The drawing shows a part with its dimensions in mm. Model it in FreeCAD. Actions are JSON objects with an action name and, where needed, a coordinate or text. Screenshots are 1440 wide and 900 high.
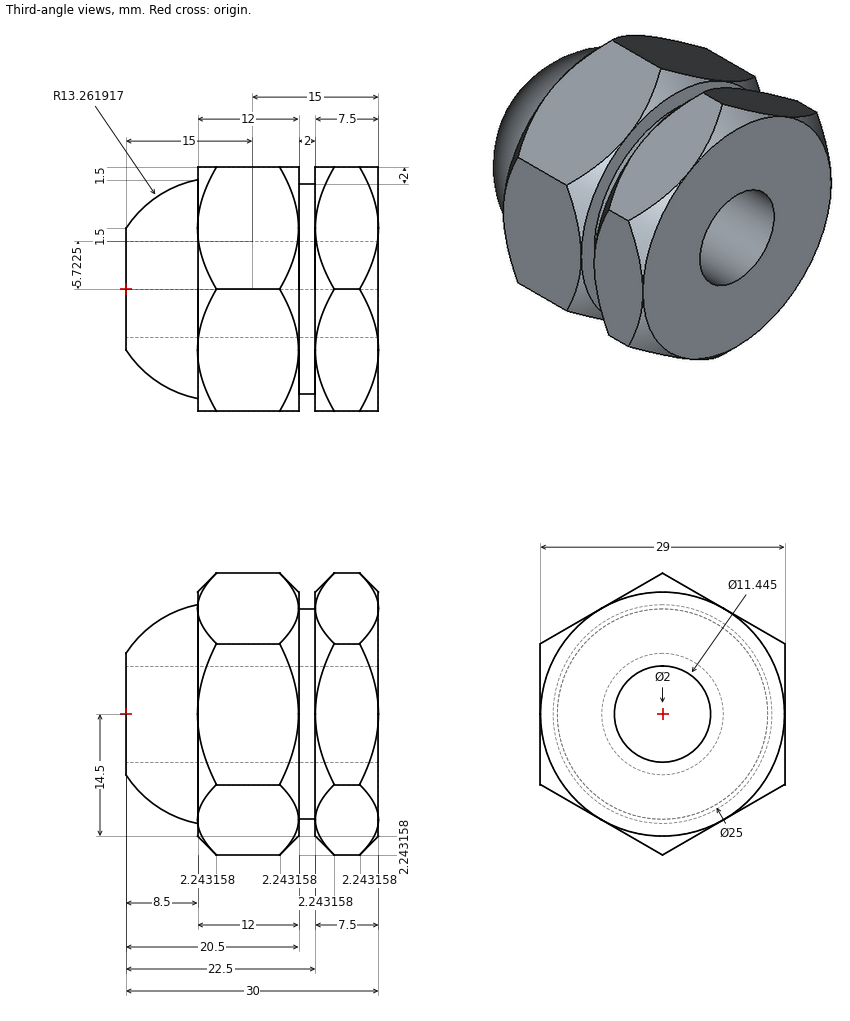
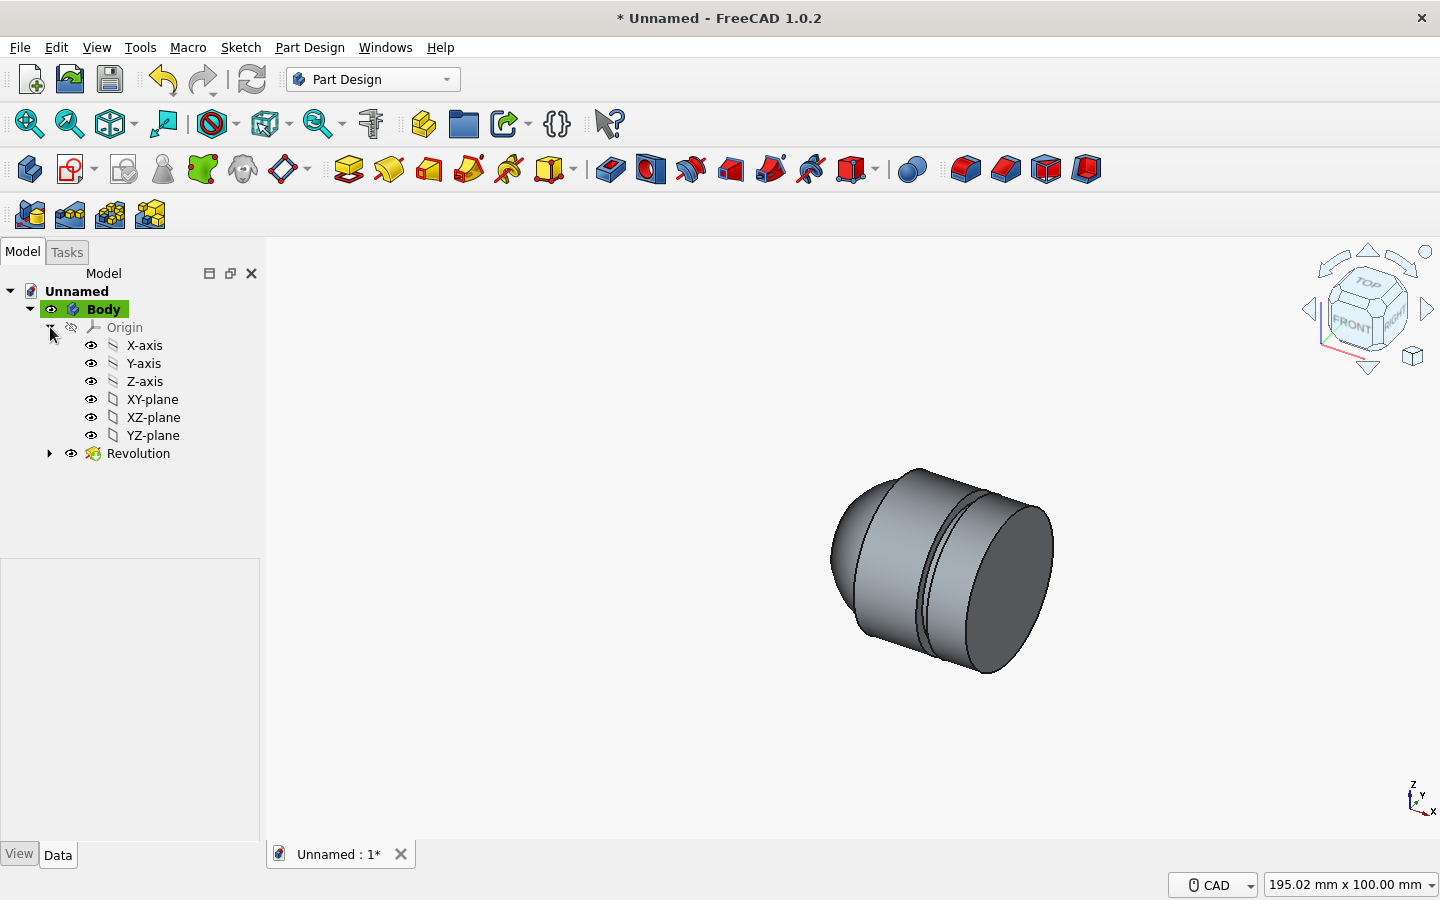
{"action": "left_click", "coordinate": [136, 435]}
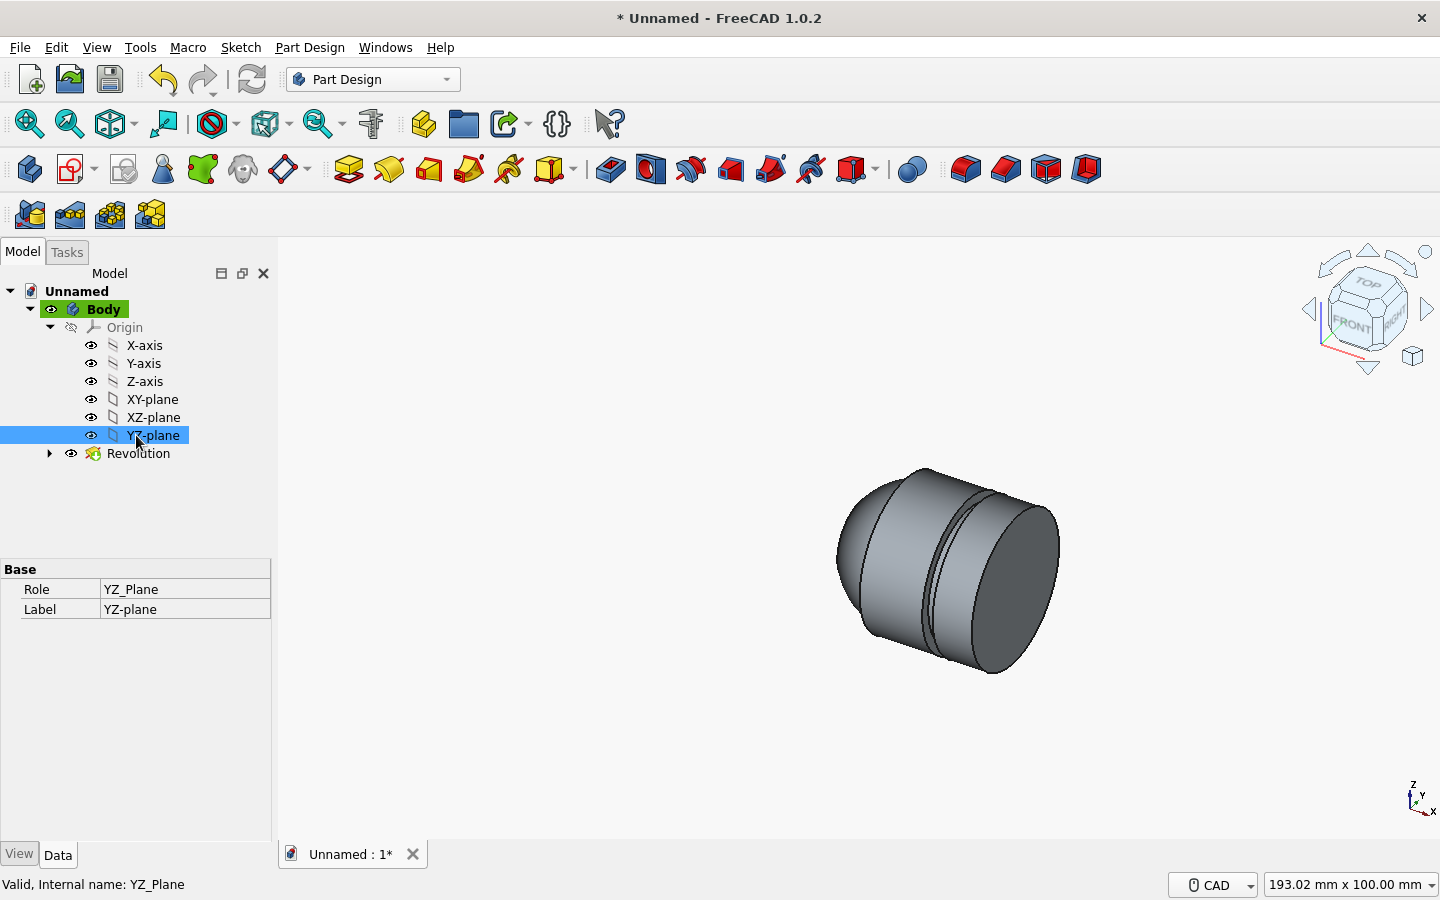
{"action": "left_click", "coordinate": [284, 170]}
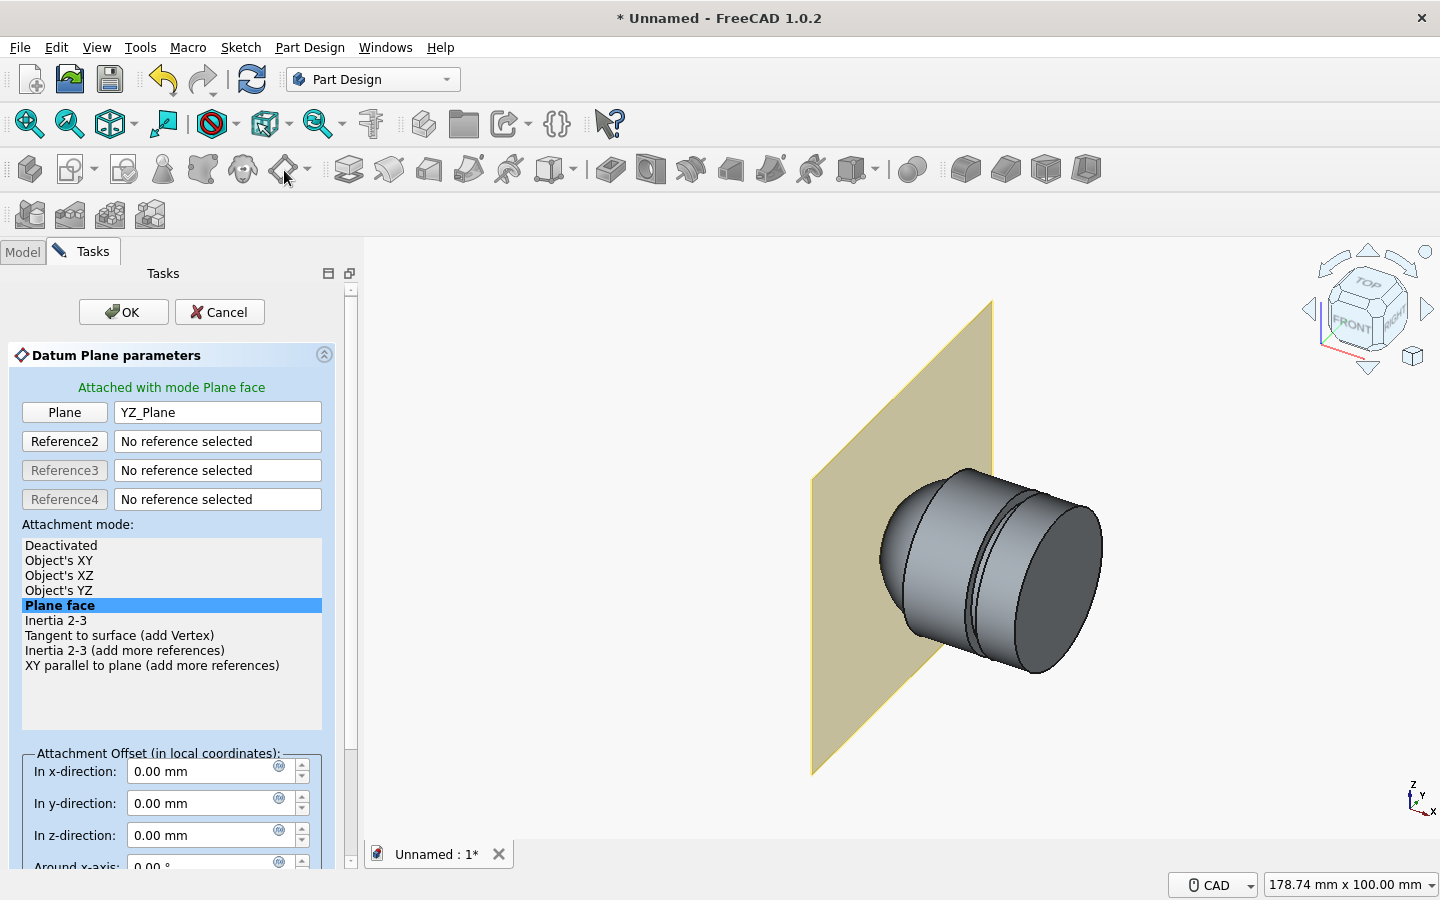
{"action": "triple_click", "coordinate": [210, 835]}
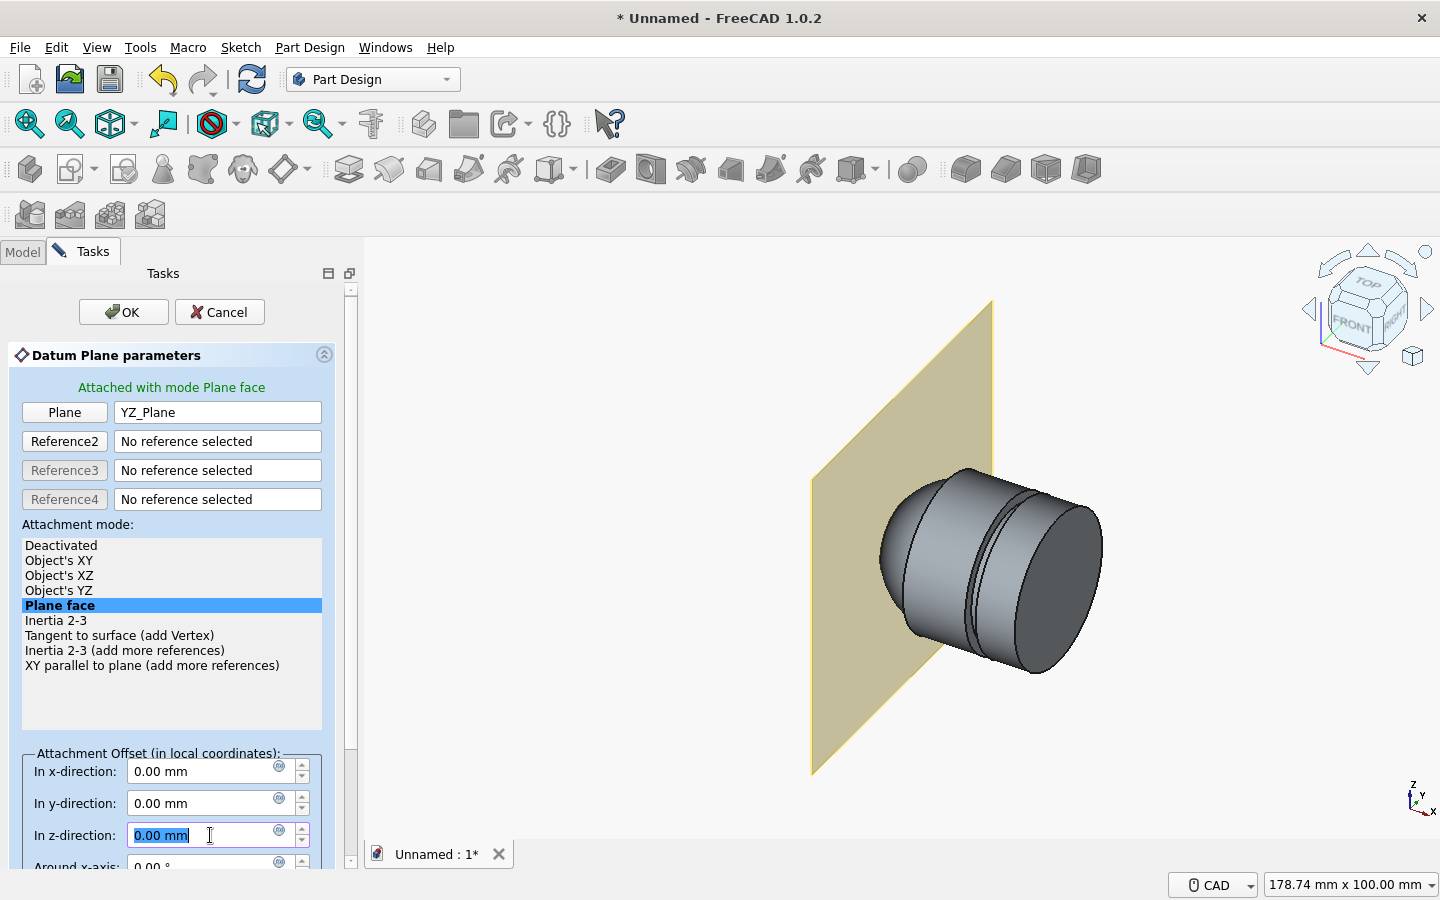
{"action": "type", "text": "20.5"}
{"action": "key", "text": "Tab"}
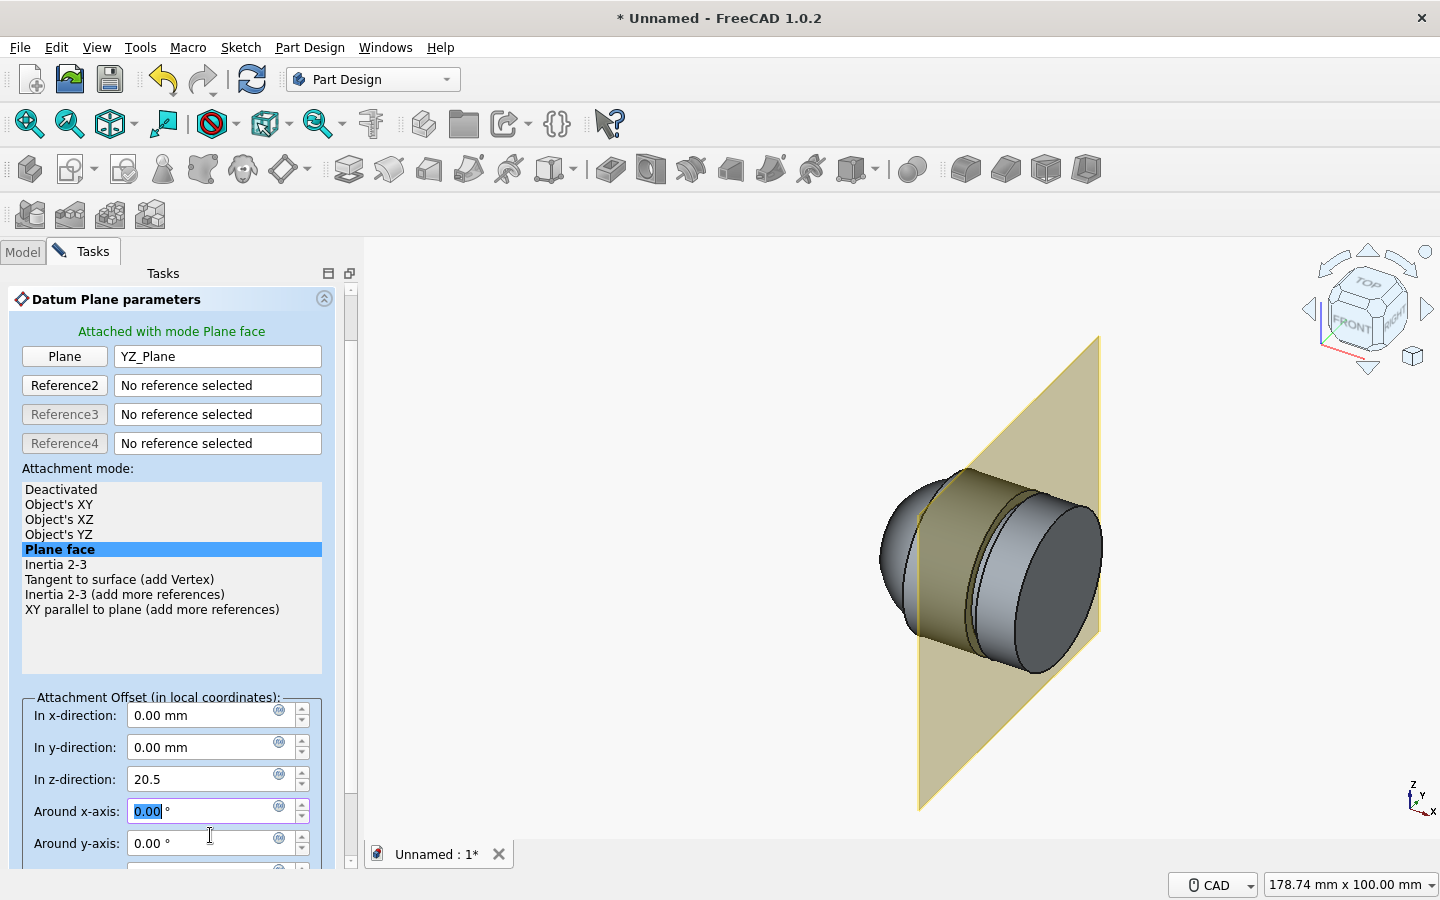
{"action": "scroll", "coordinate": [351, 576], "scroll_direction": "up", "scroll_amount": 2}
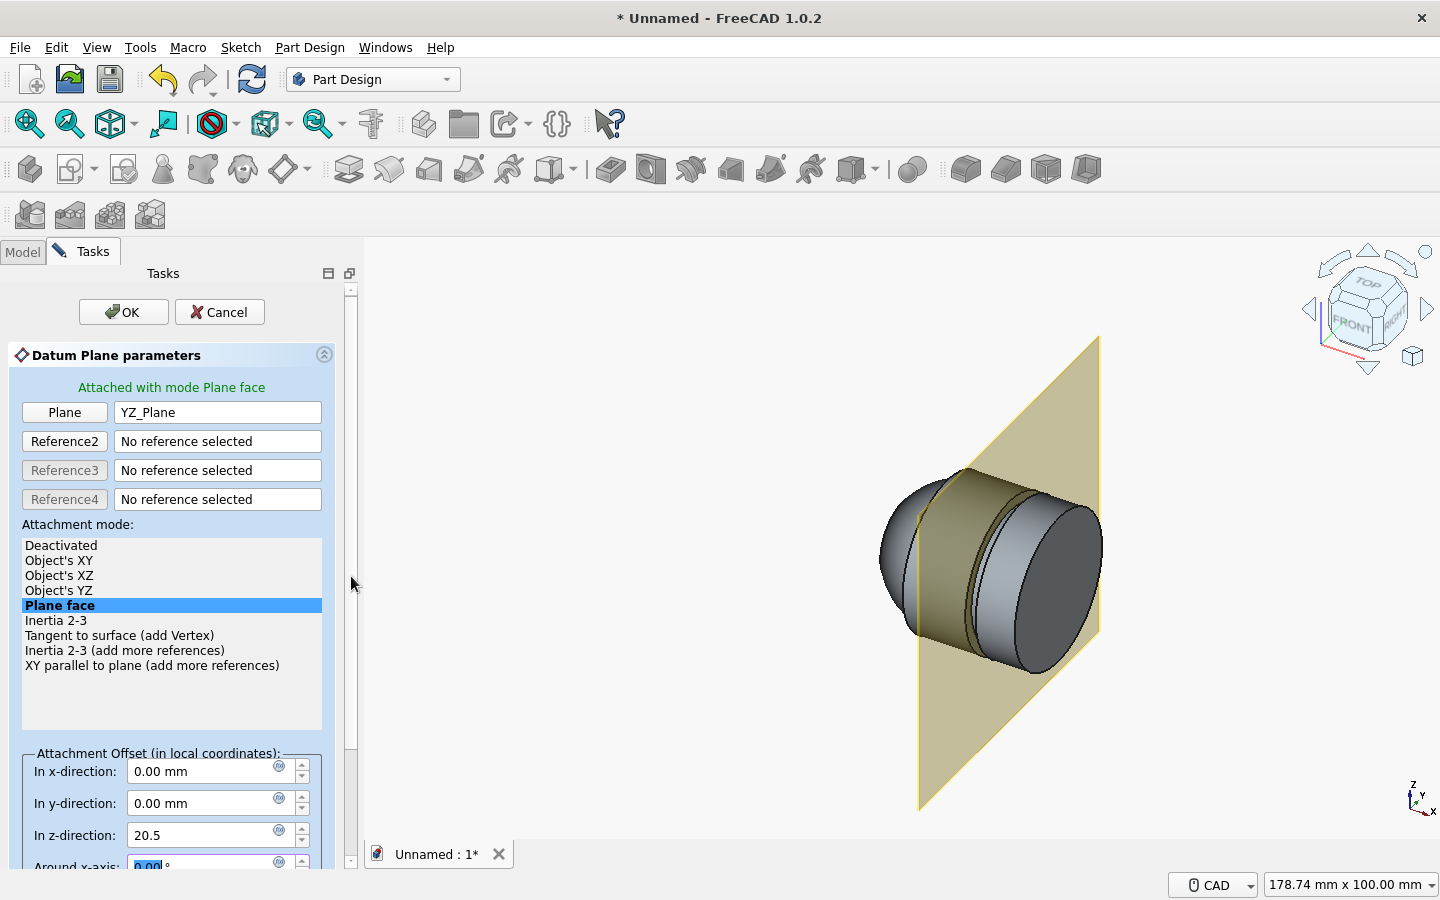
{"action": "left_click", "coordinate": [124, 312]}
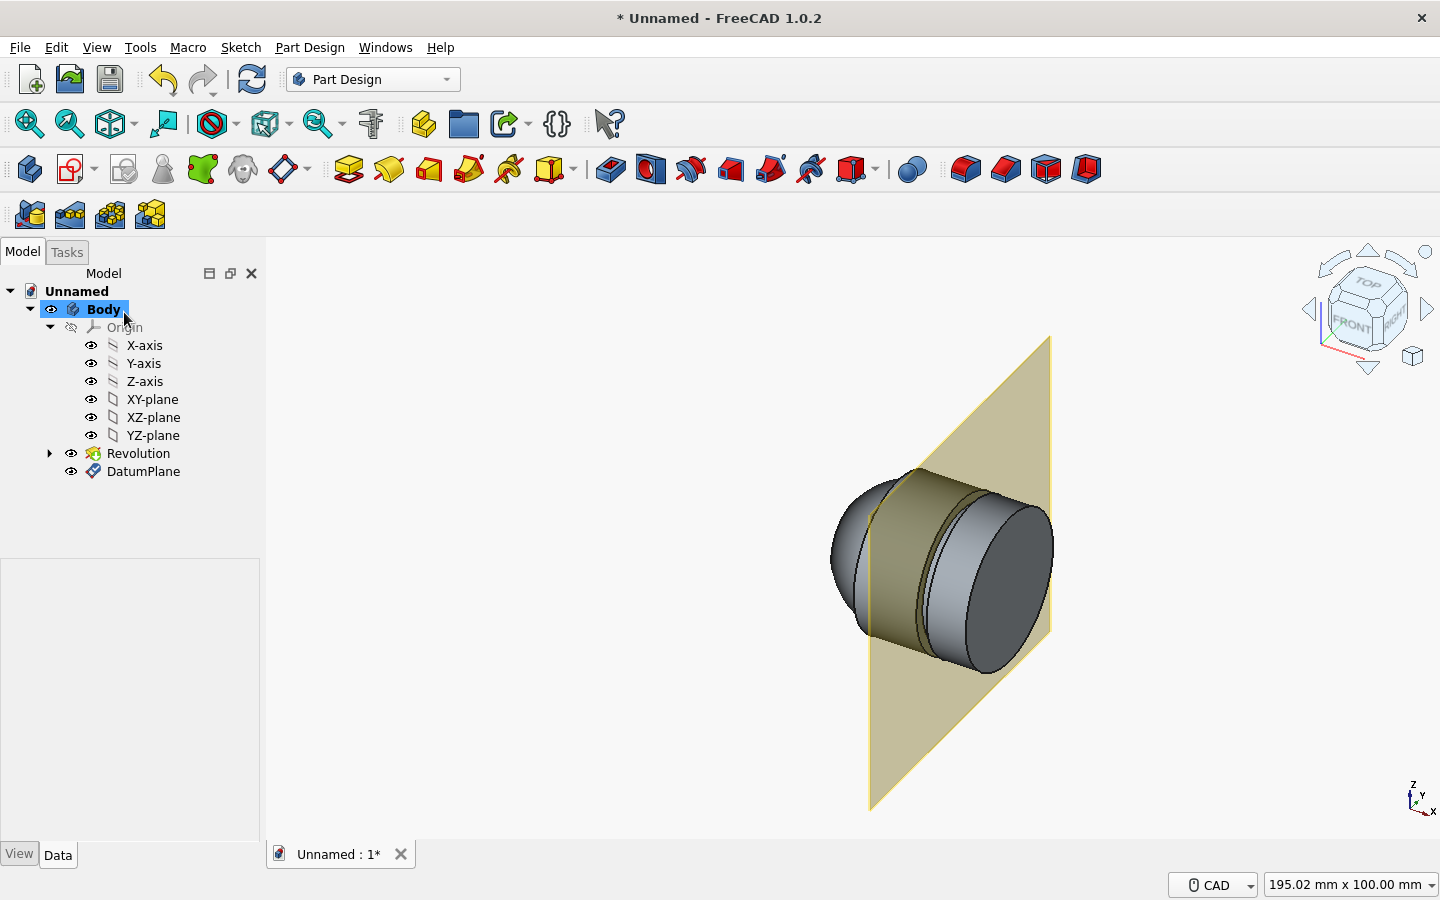
{"action": "left_click", "coordinate": [116, 471]}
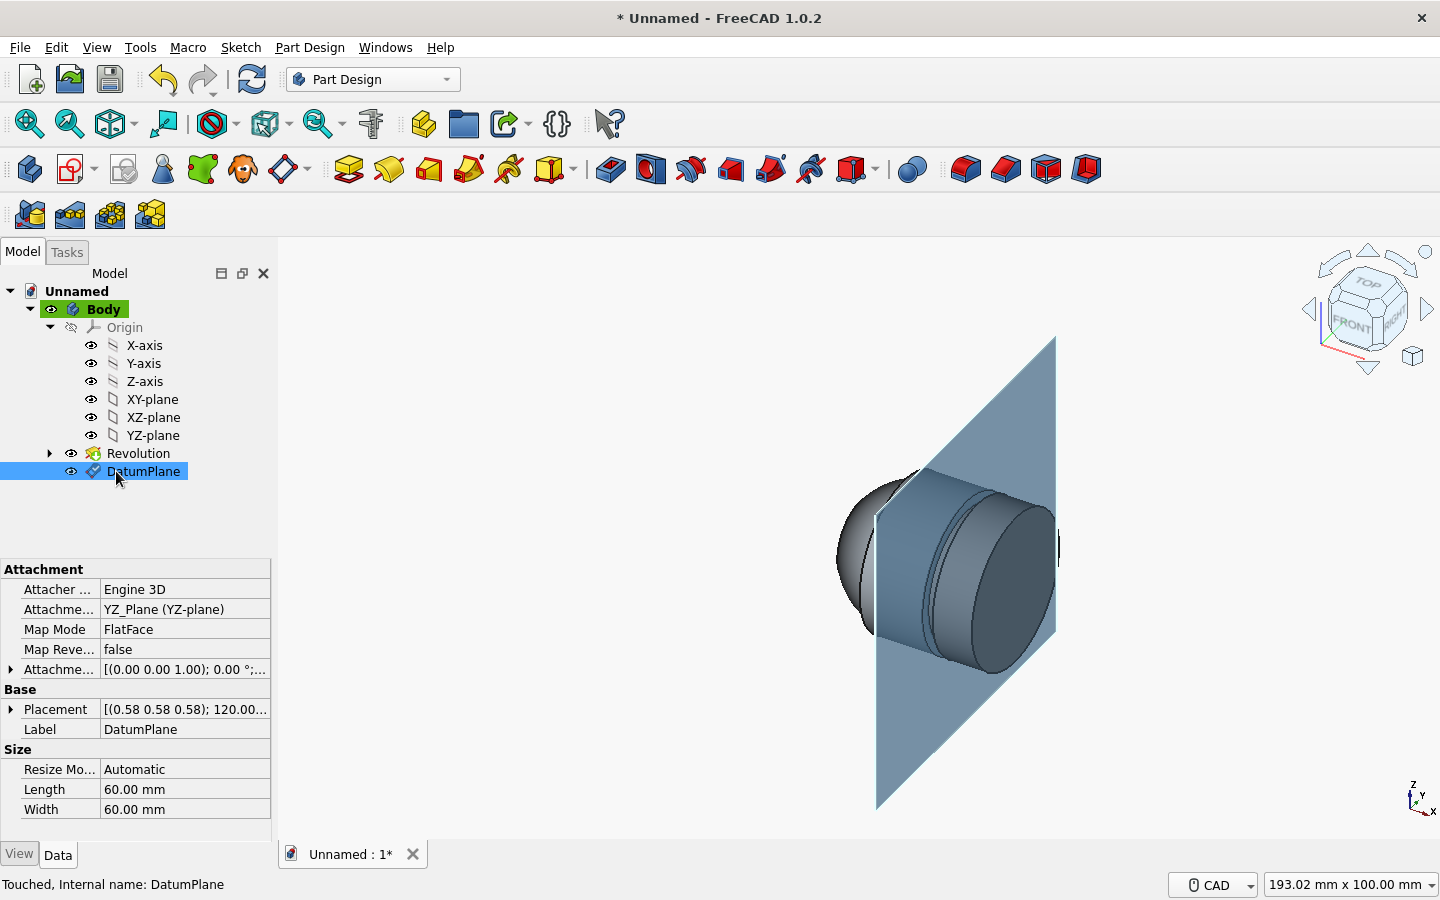
{"action": "left_click", "coordinate": [70, 170]}